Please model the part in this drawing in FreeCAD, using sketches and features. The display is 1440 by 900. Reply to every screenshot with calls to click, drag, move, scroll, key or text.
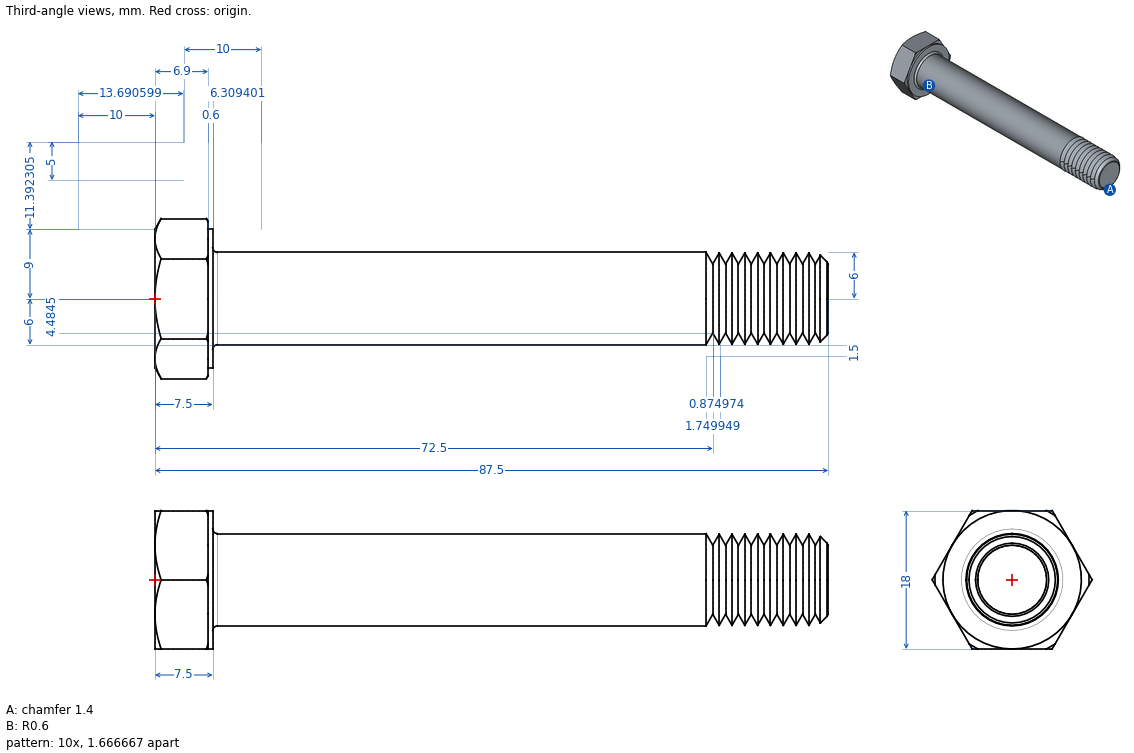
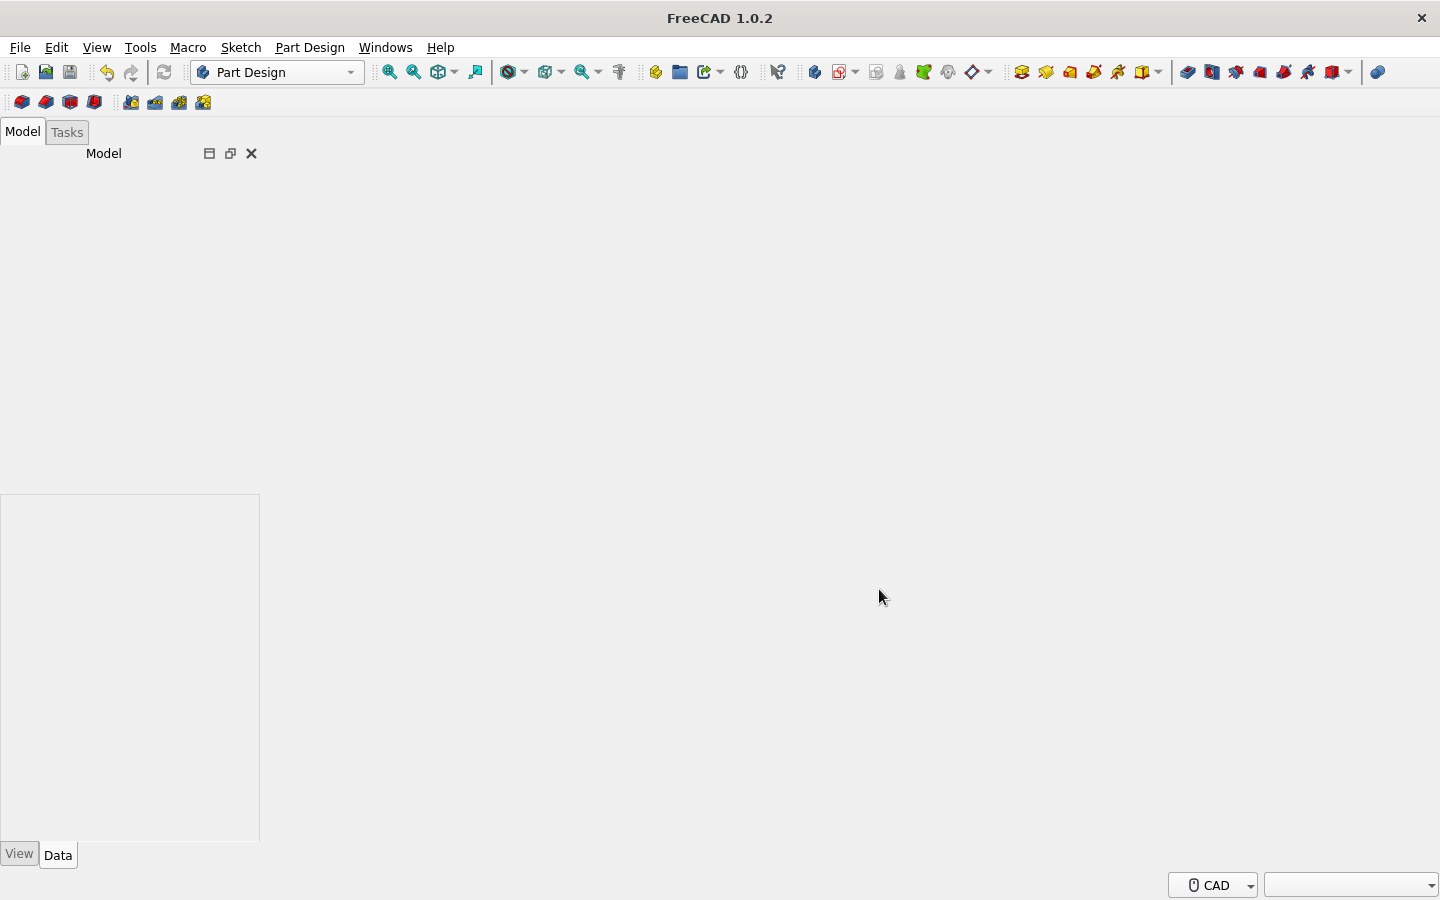
click(22, 72)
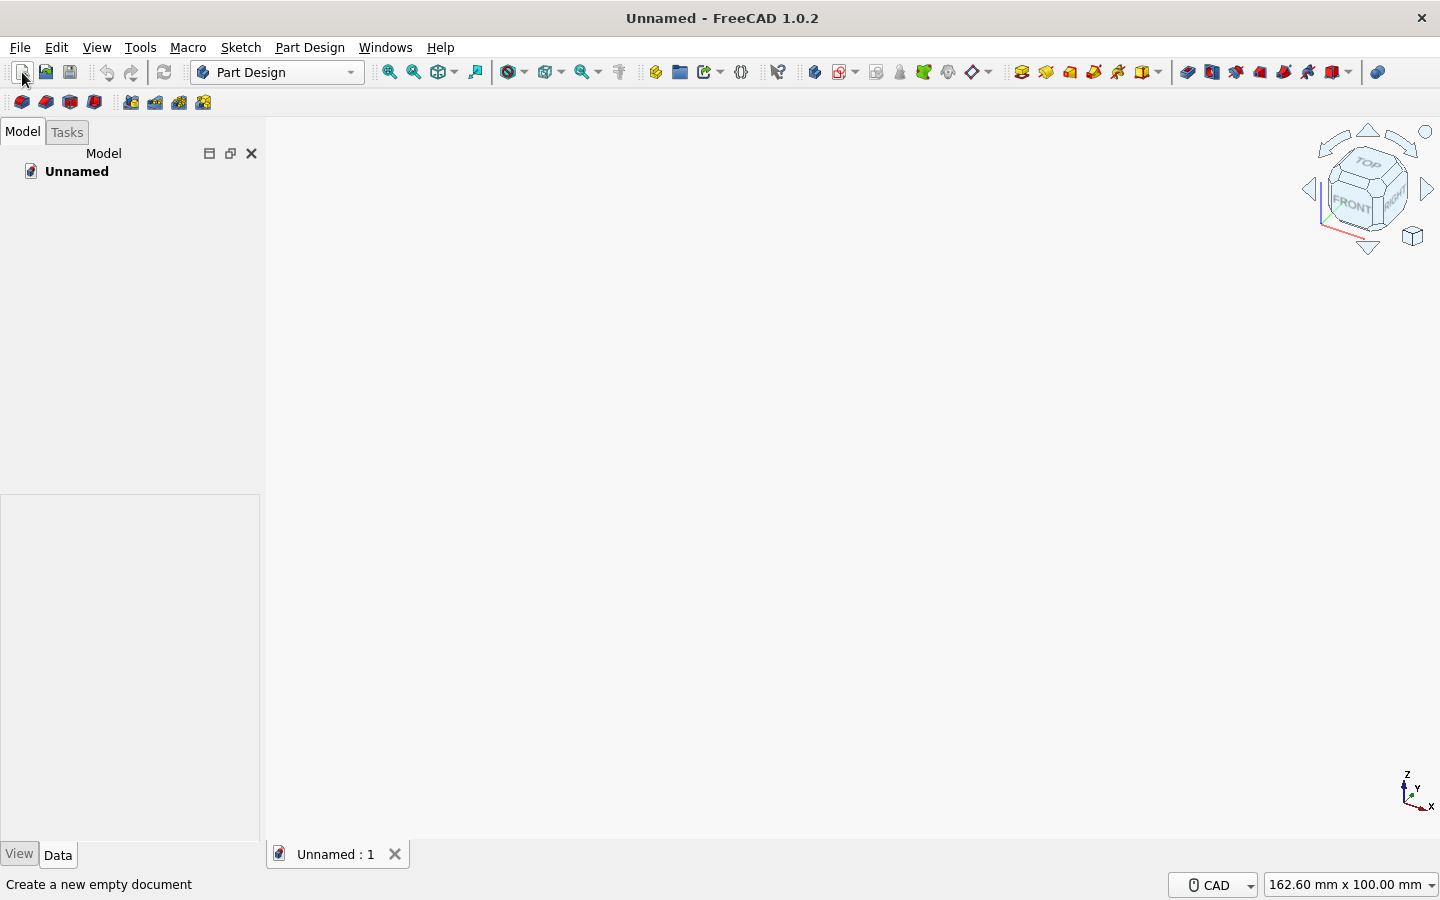
click(840, 72)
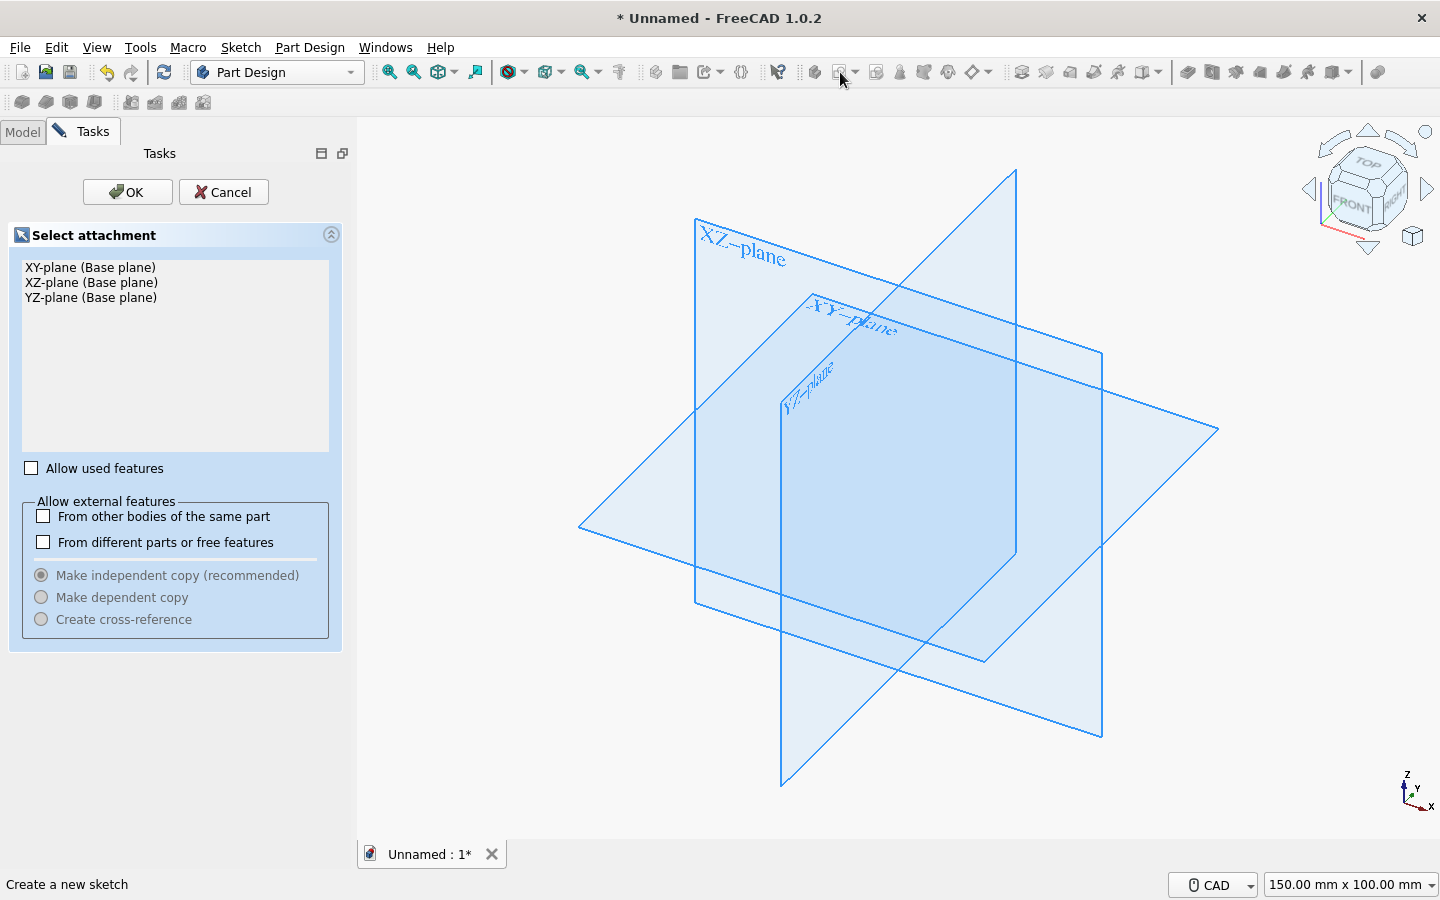
click(82, 298)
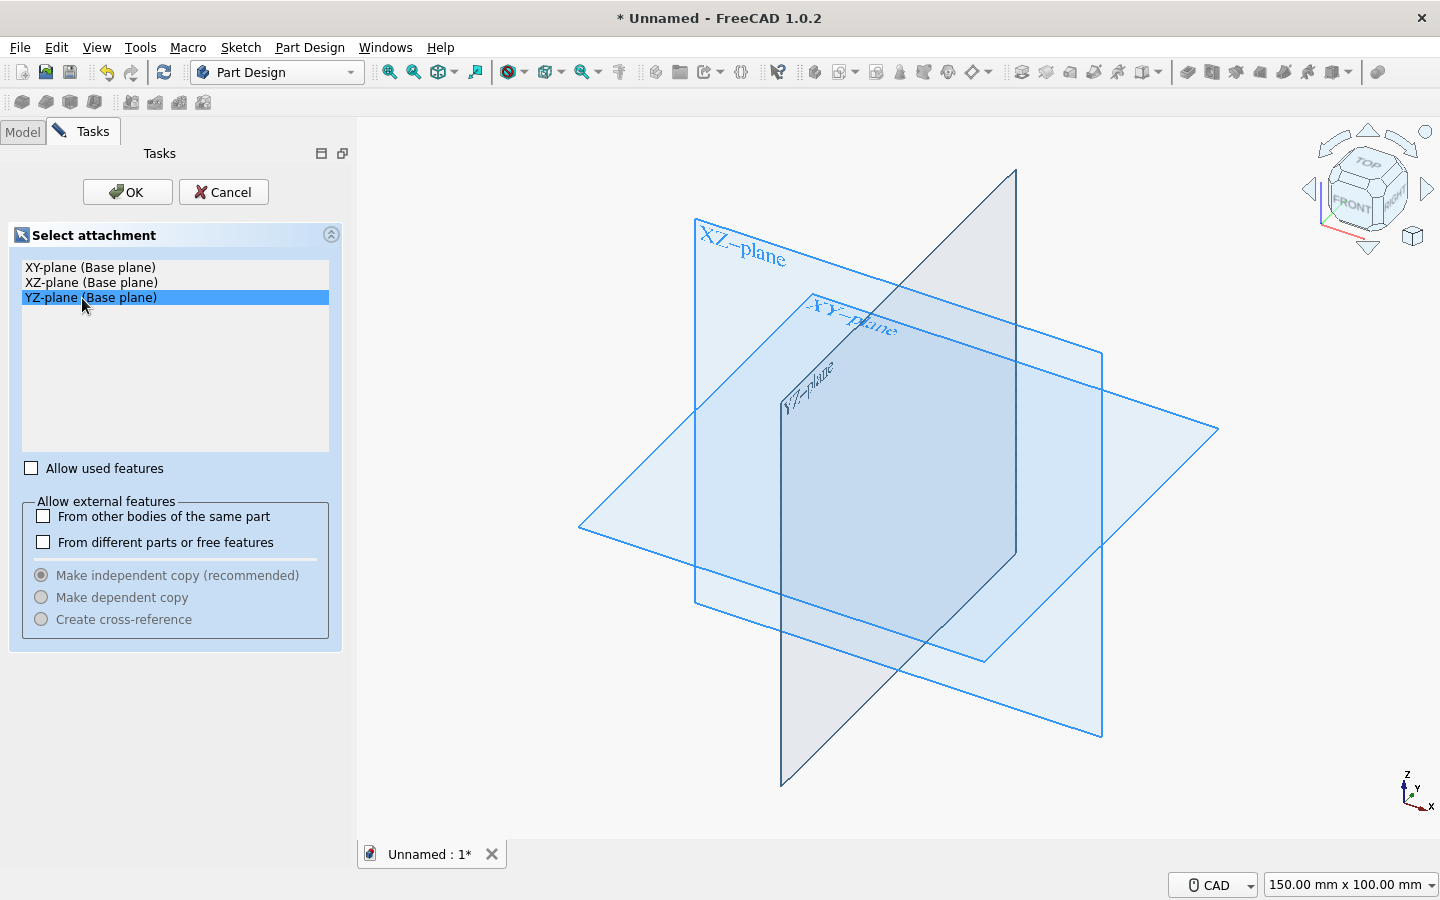
click(128, 192)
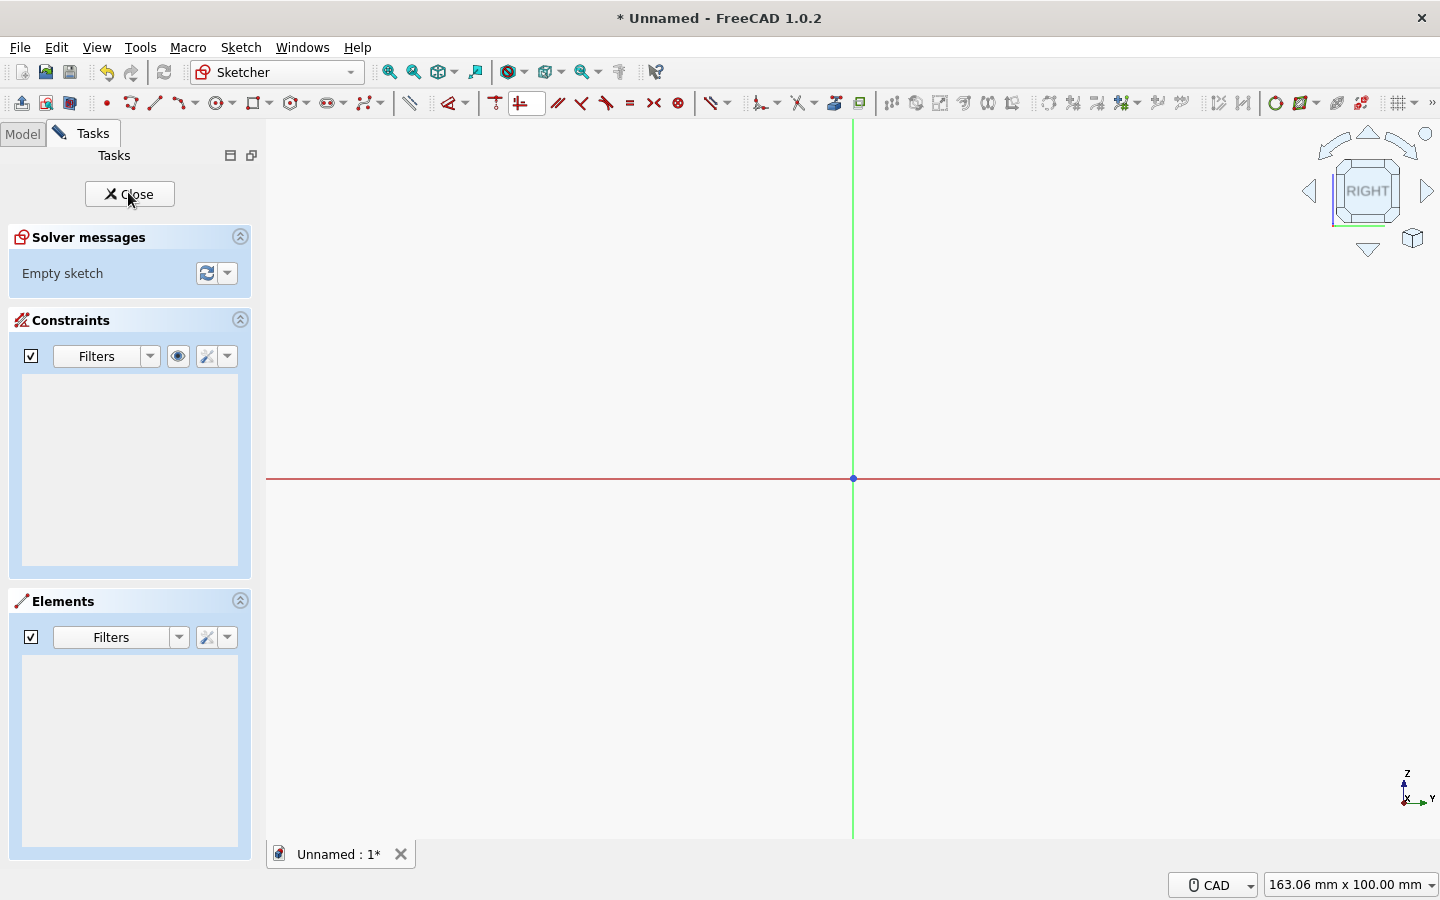
scroll(883, 479, up, 6)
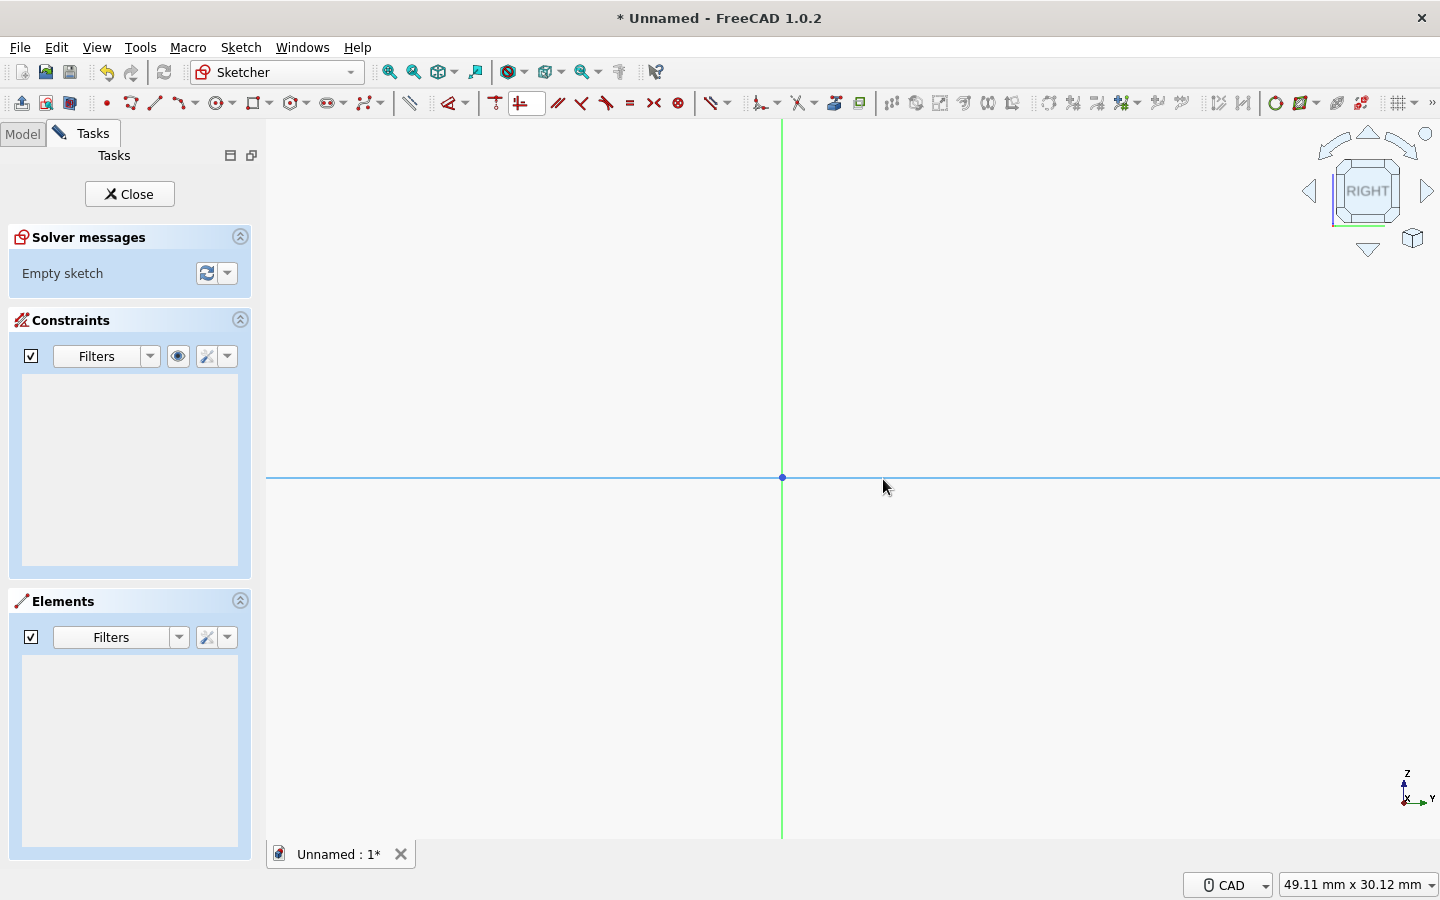
click(290, 104)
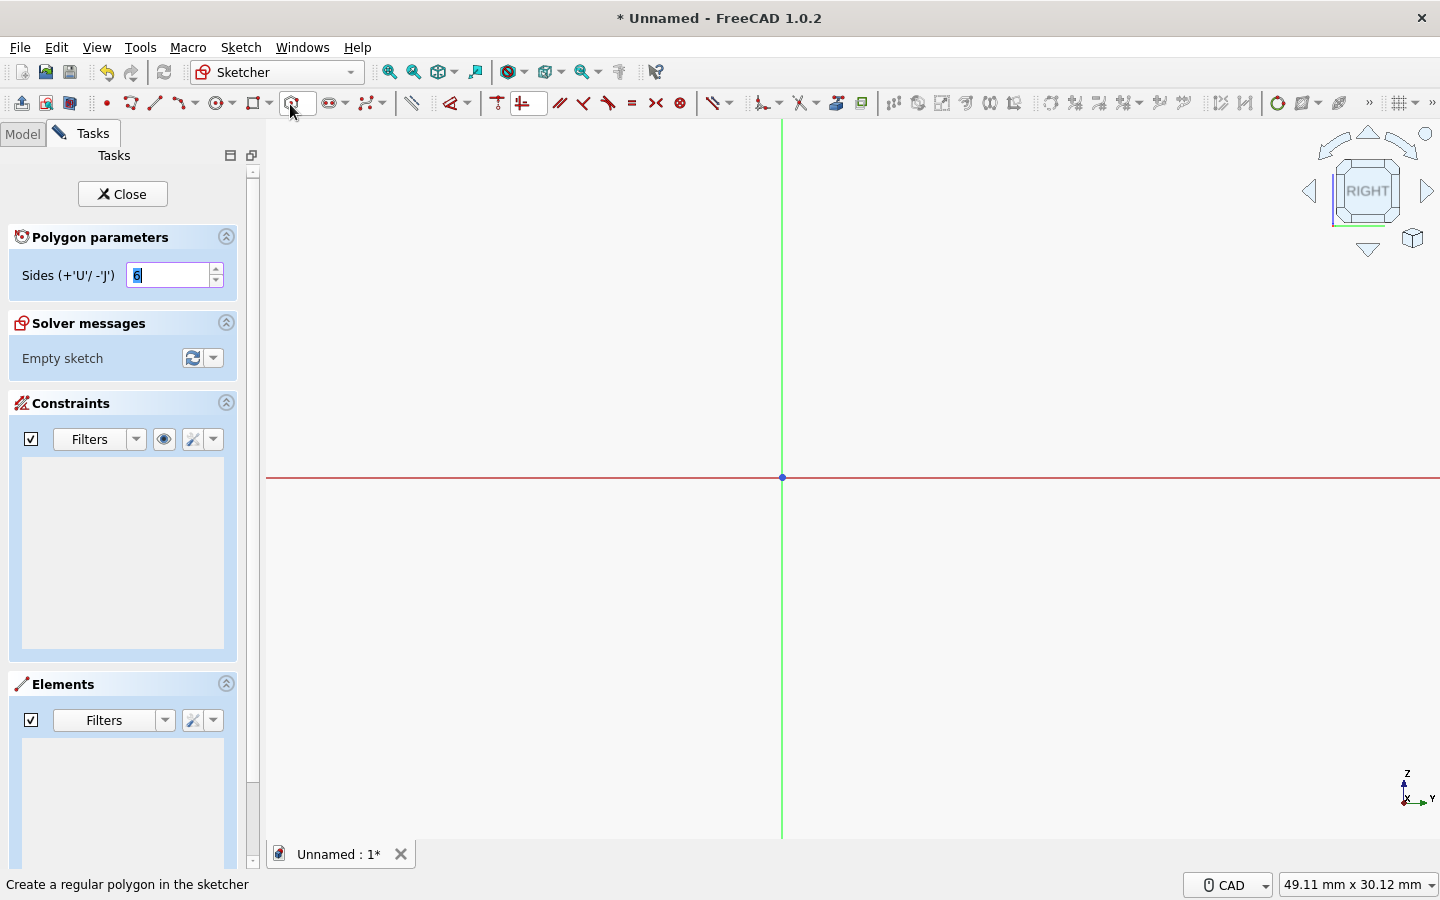
click(782, 478)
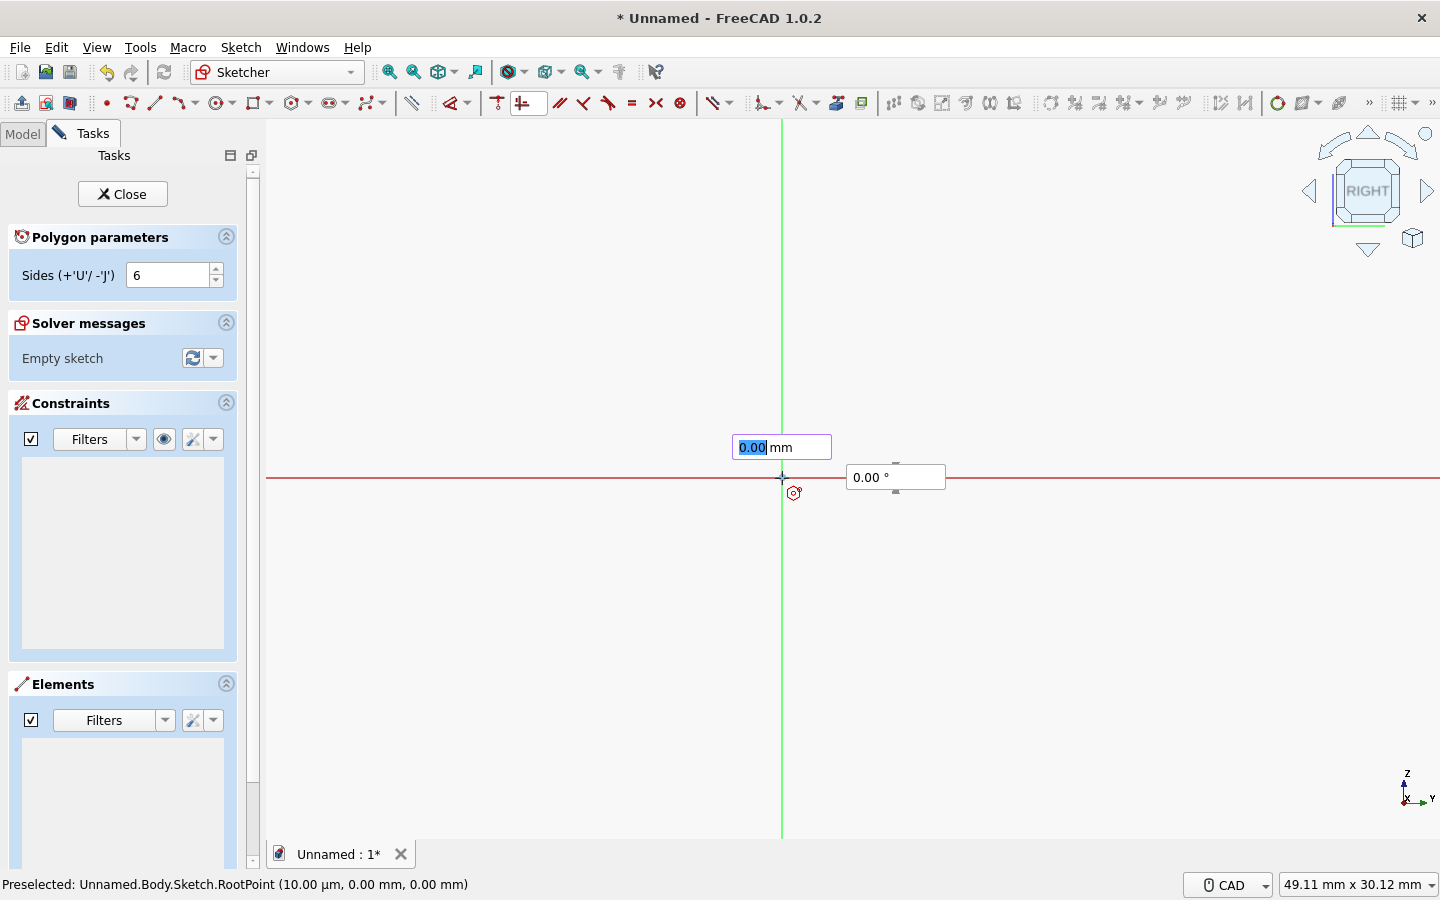
click(1031, 478)
right_click(1031, 478)